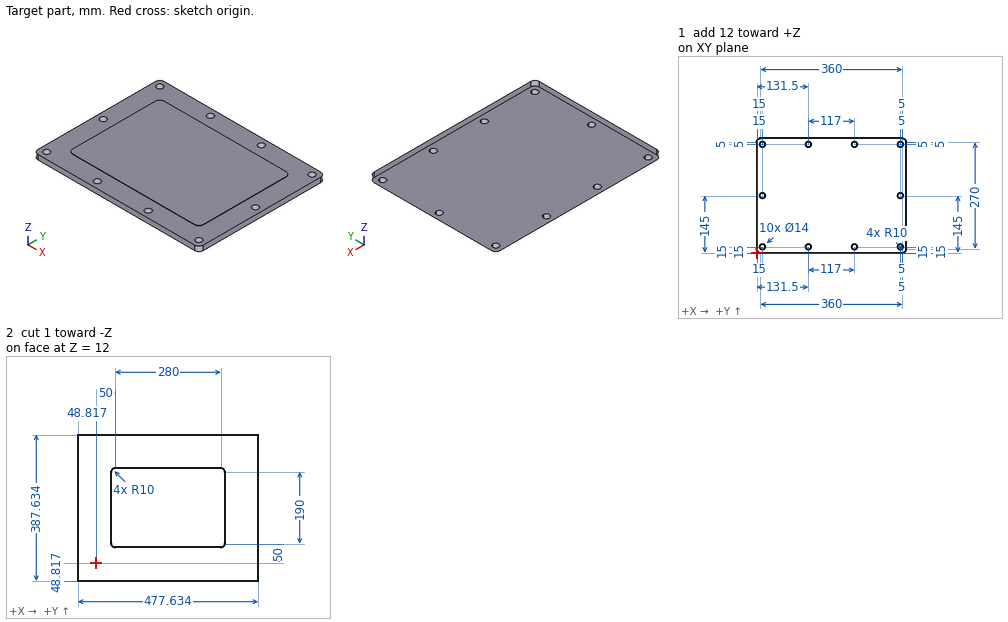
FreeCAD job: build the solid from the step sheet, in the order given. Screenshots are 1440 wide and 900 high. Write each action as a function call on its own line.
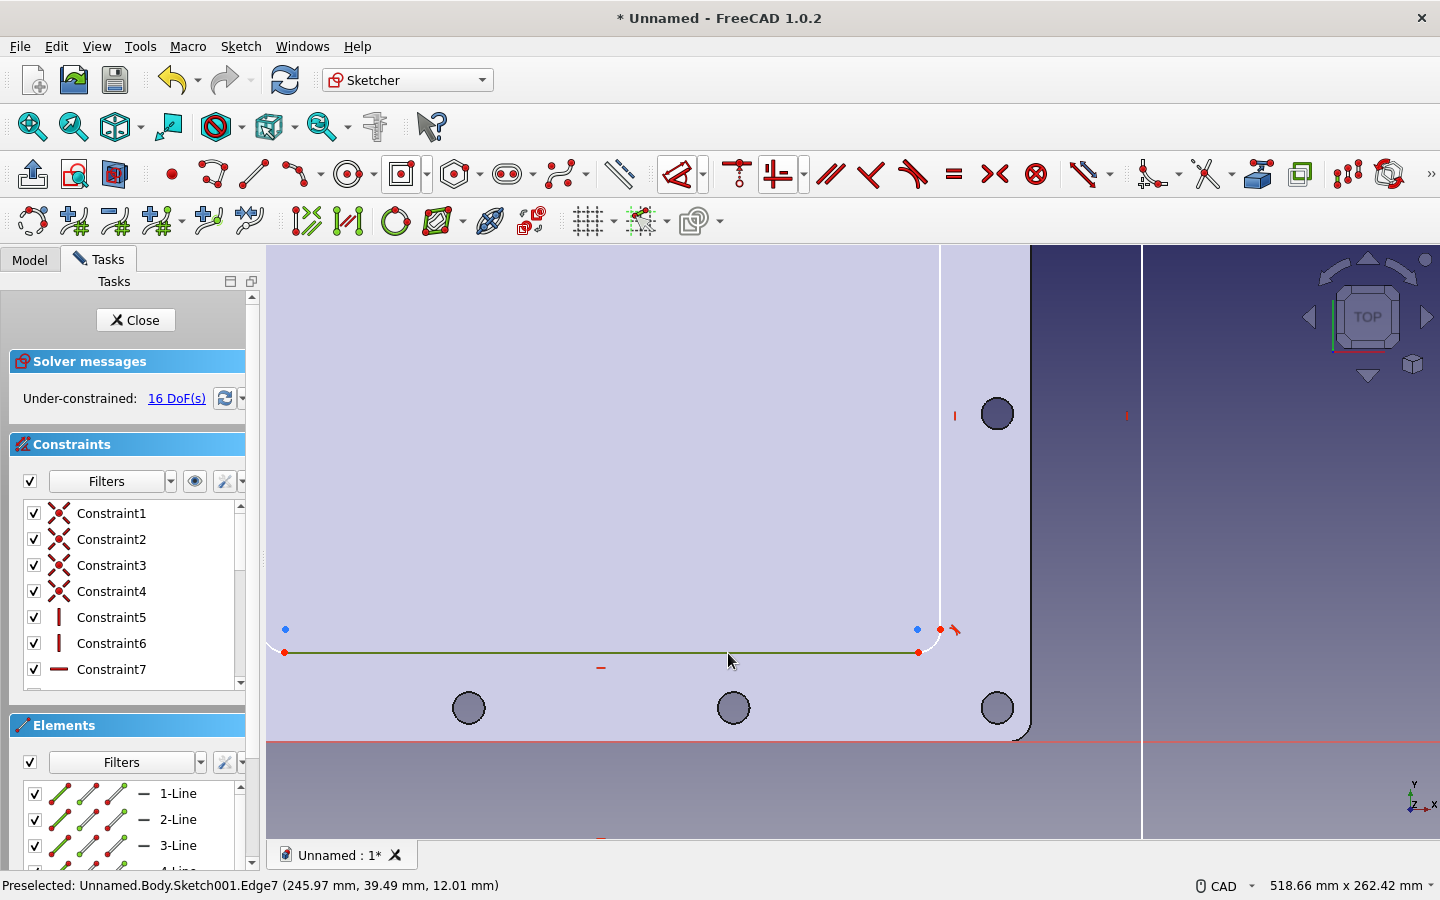
scroll(928, 650, up, 2)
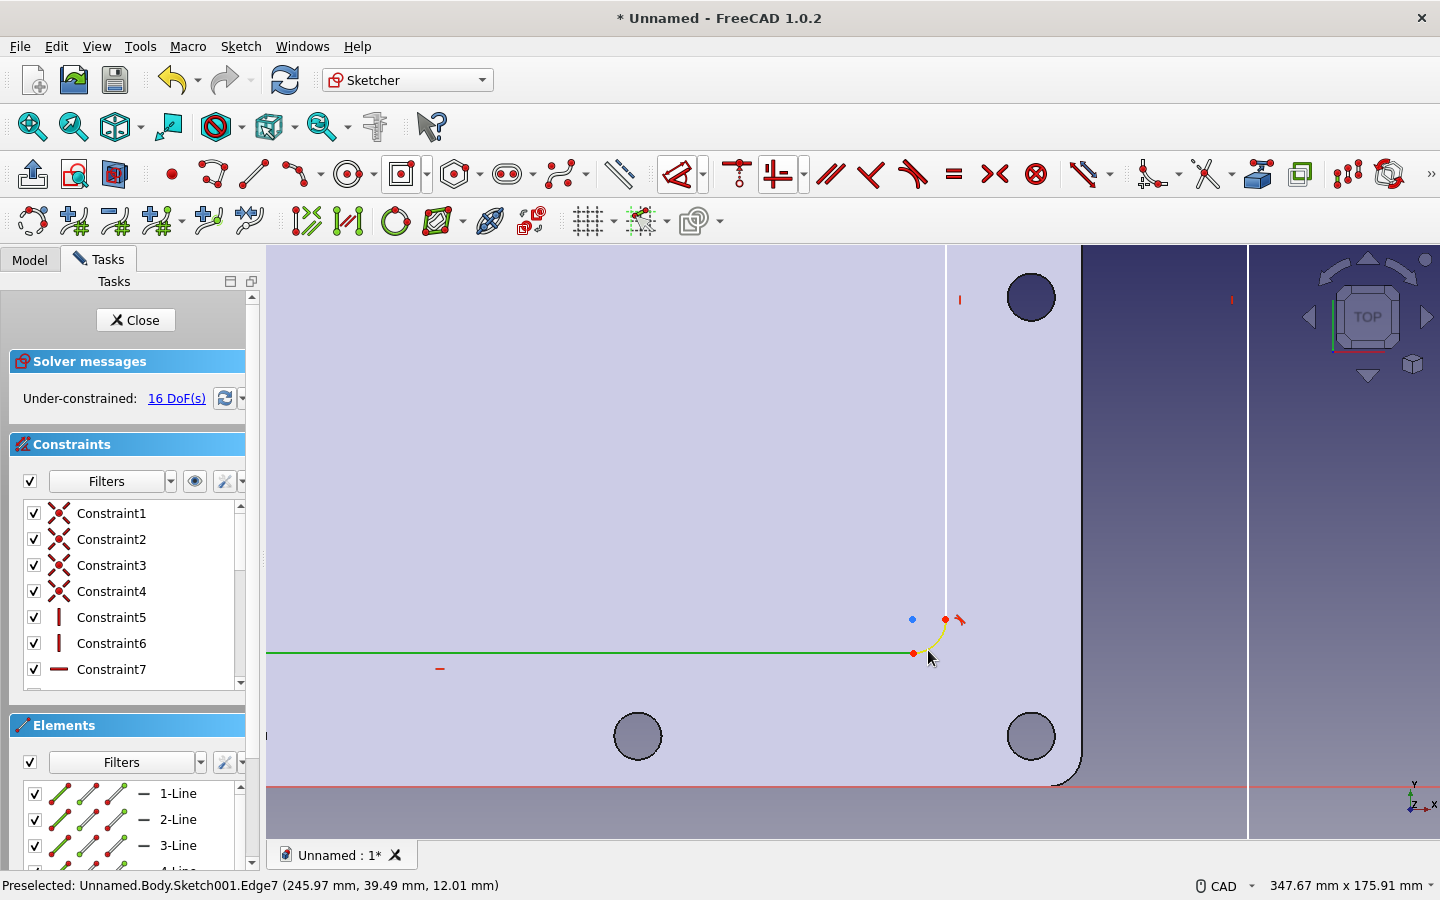
click(928, 649)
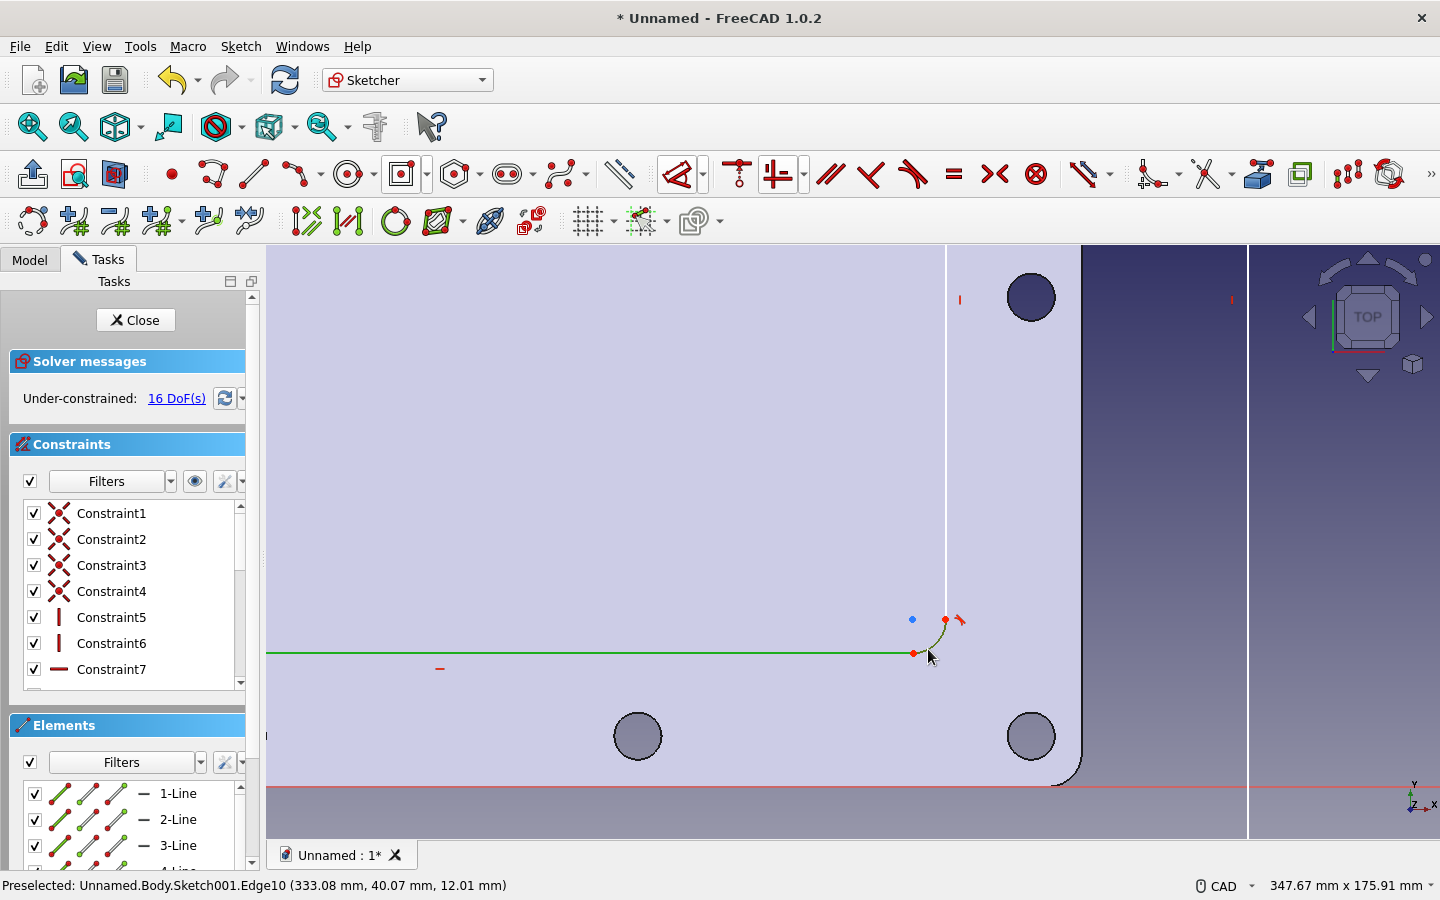
click(913, 174)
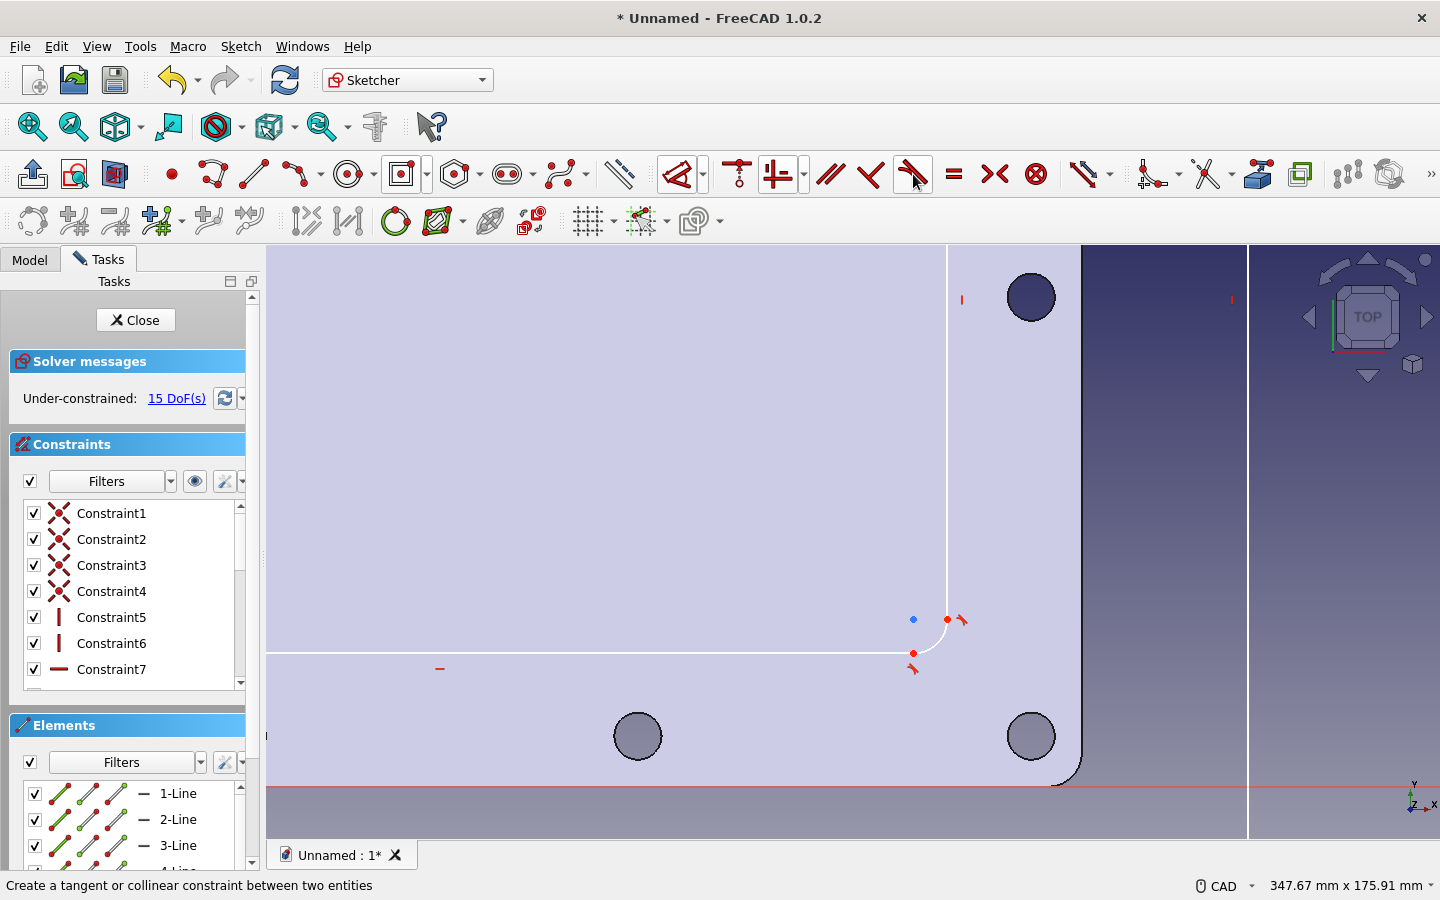
click(630, 653)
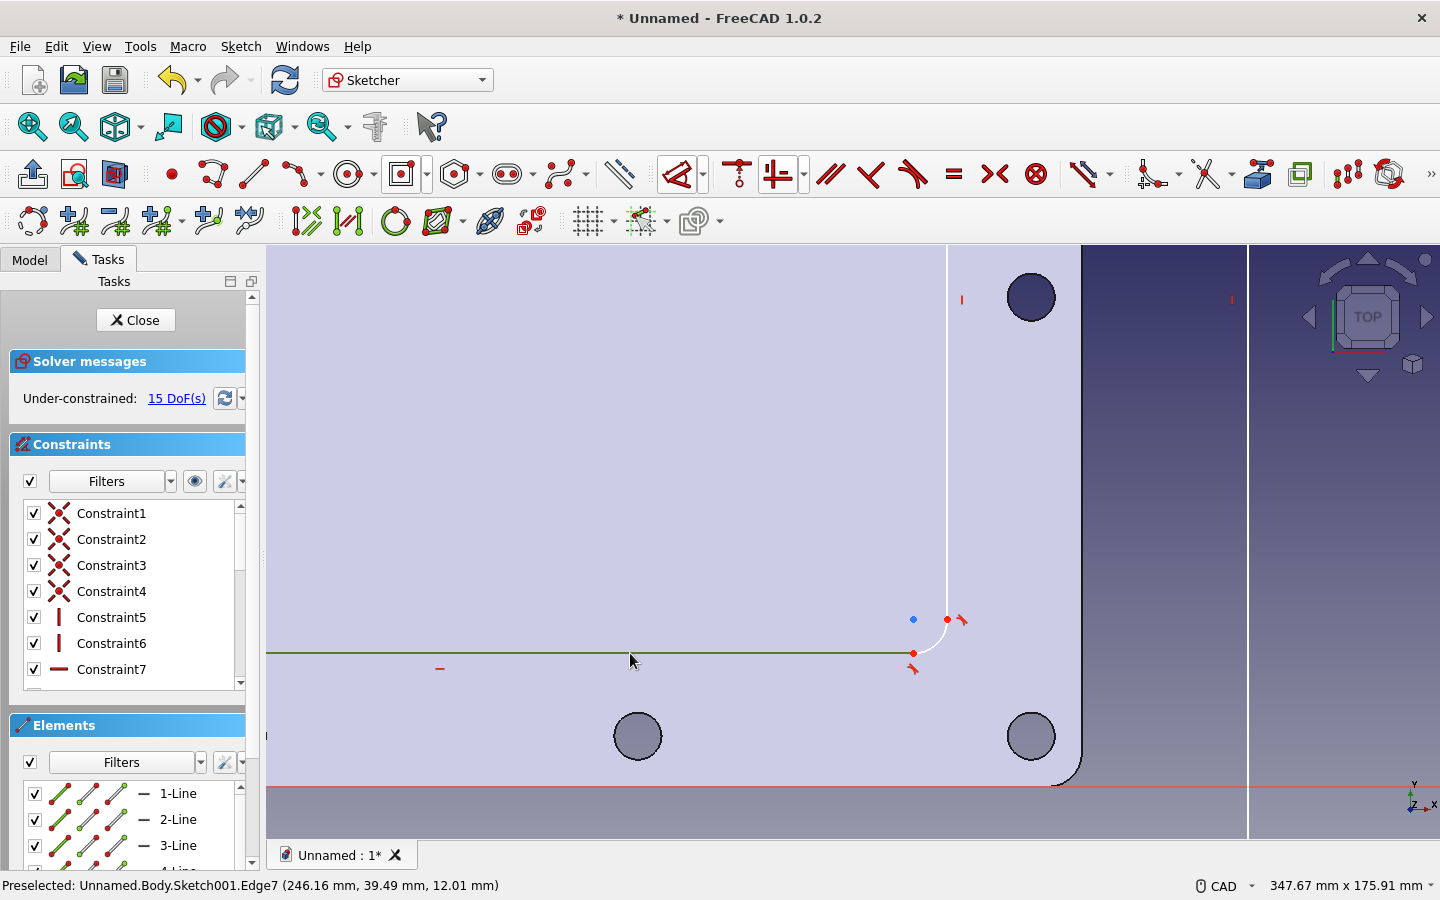
scroll(933, 648, down, 6)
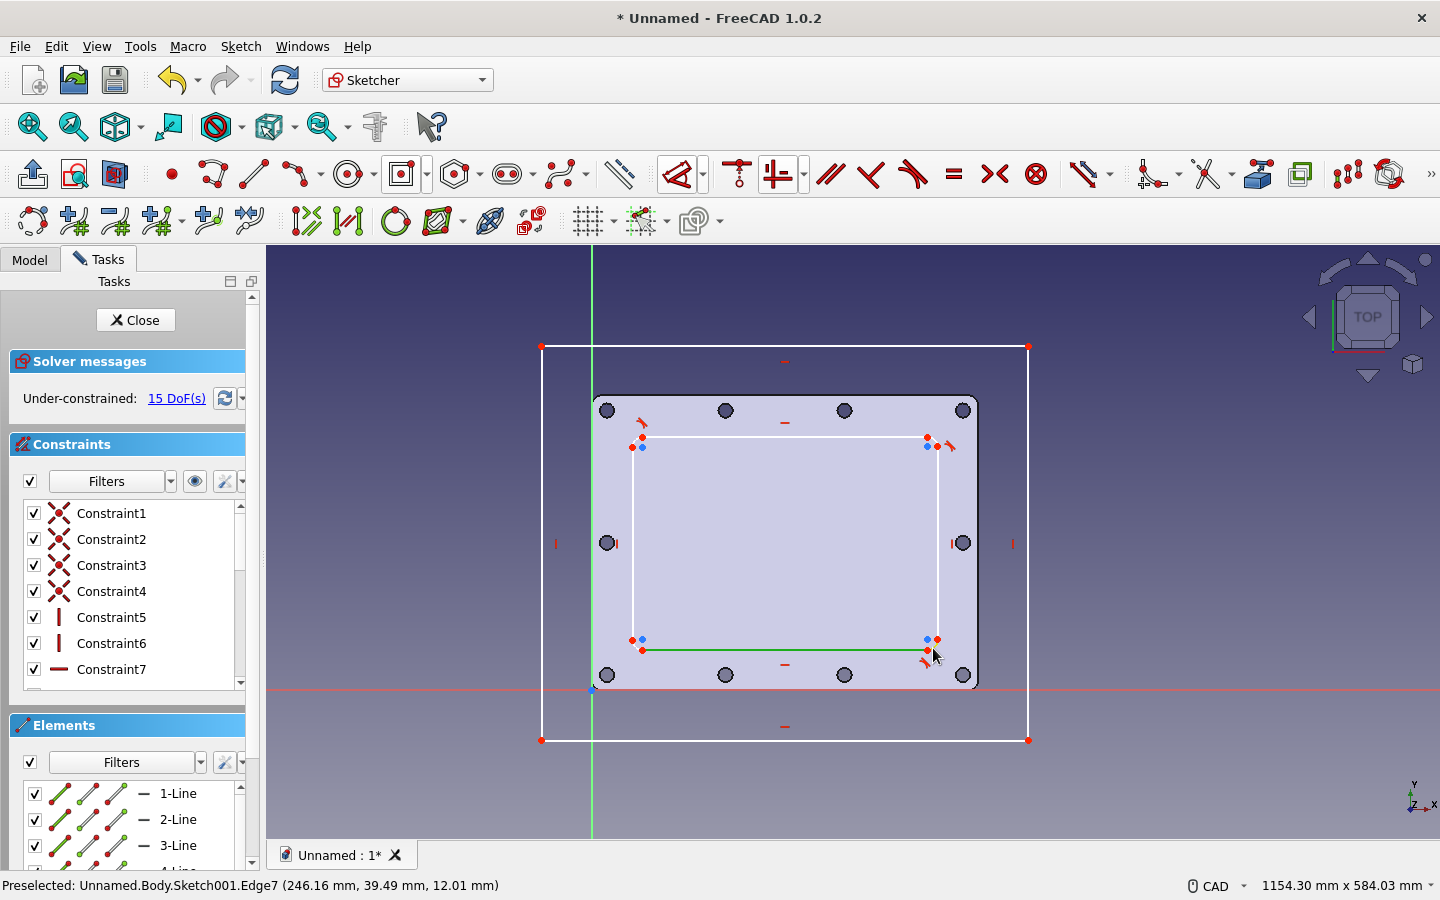
scroll(634, 645, up, 6)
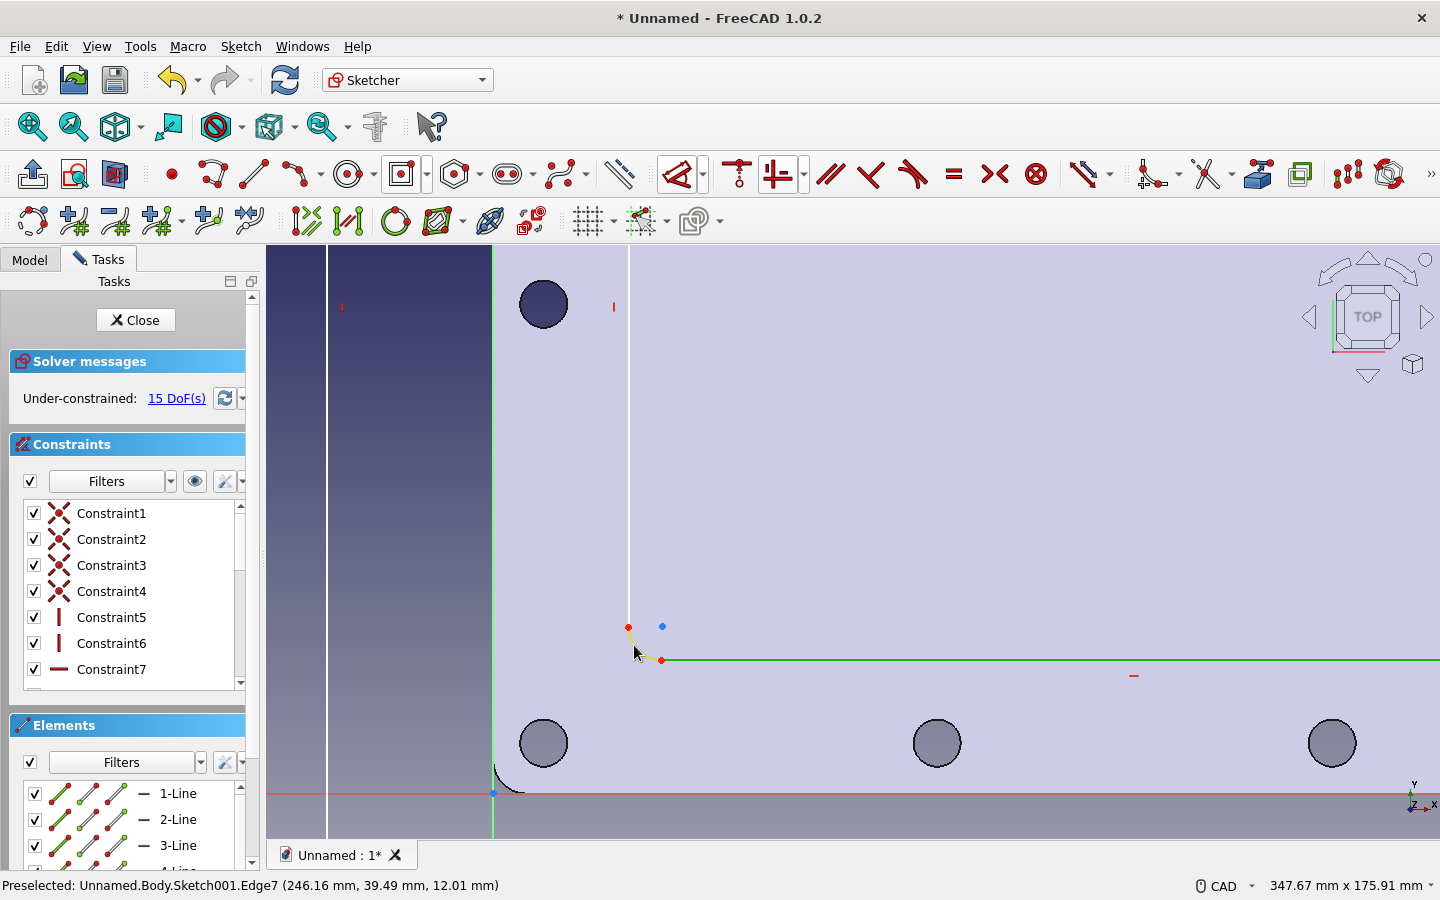
click(633, 642)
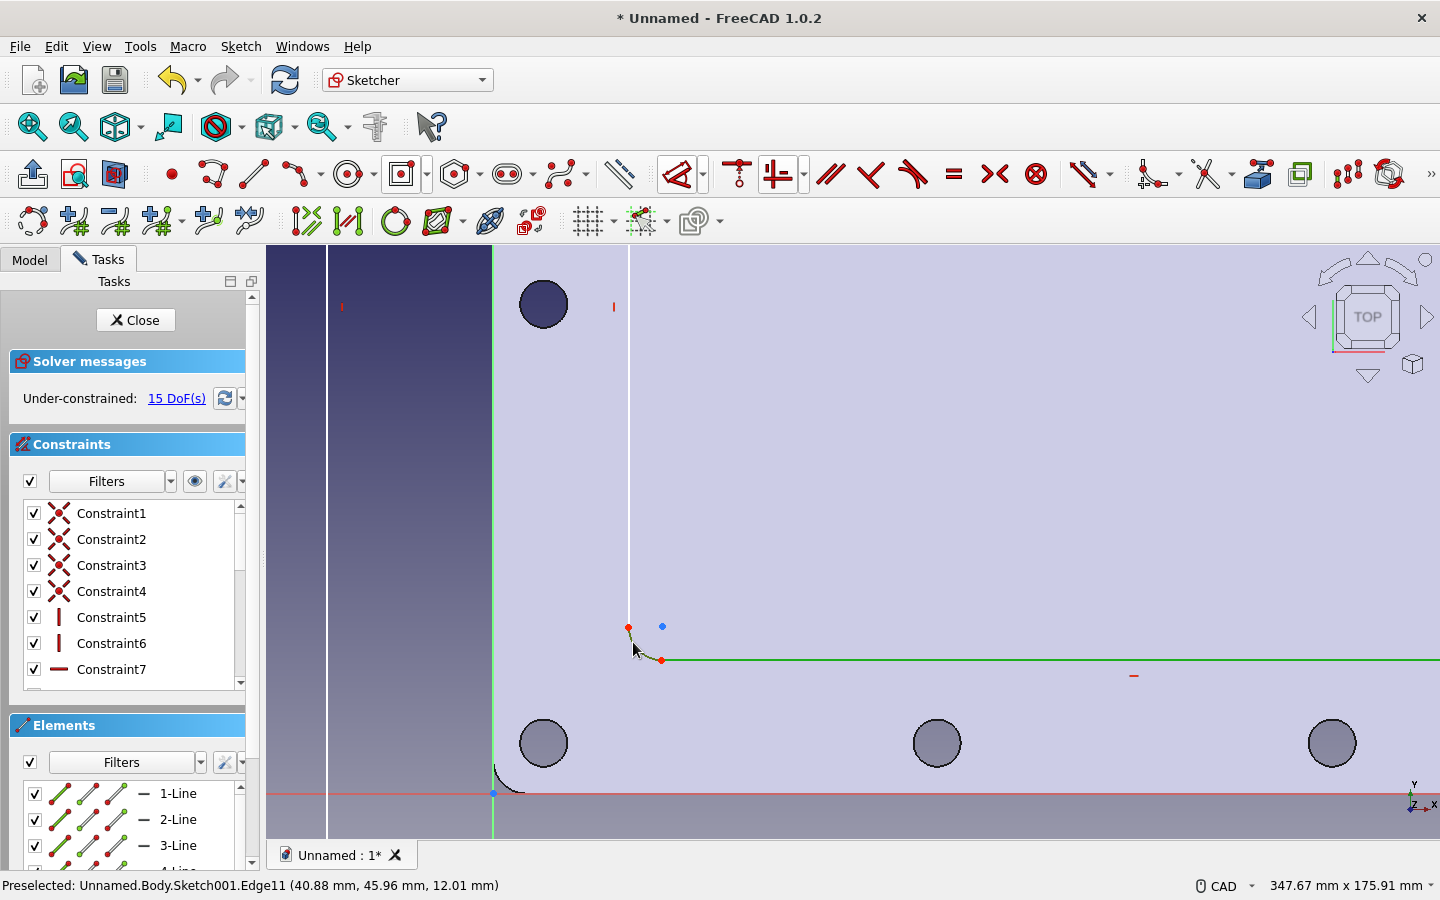
click(913, 174)